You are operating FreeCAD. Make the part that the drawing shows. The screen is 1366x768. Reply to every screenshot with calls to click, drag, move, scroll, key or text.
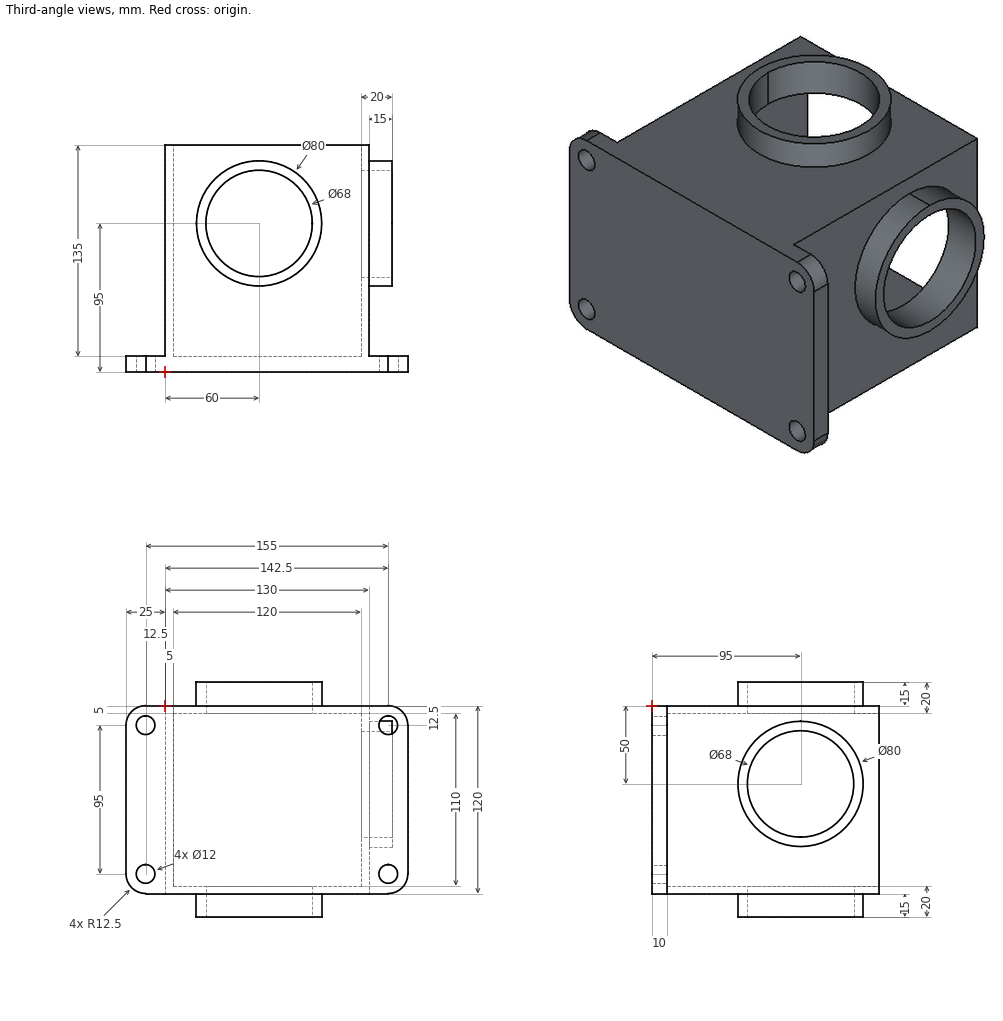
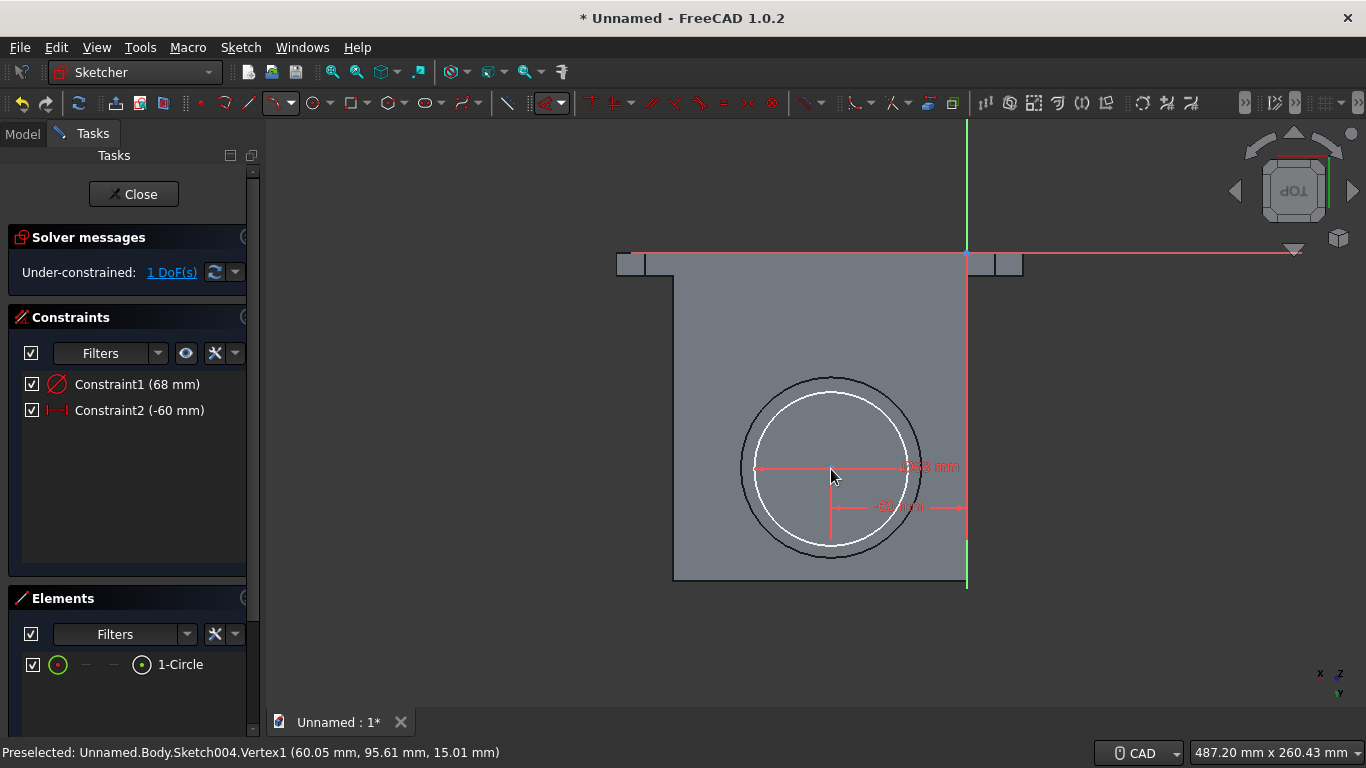
click(831, 469)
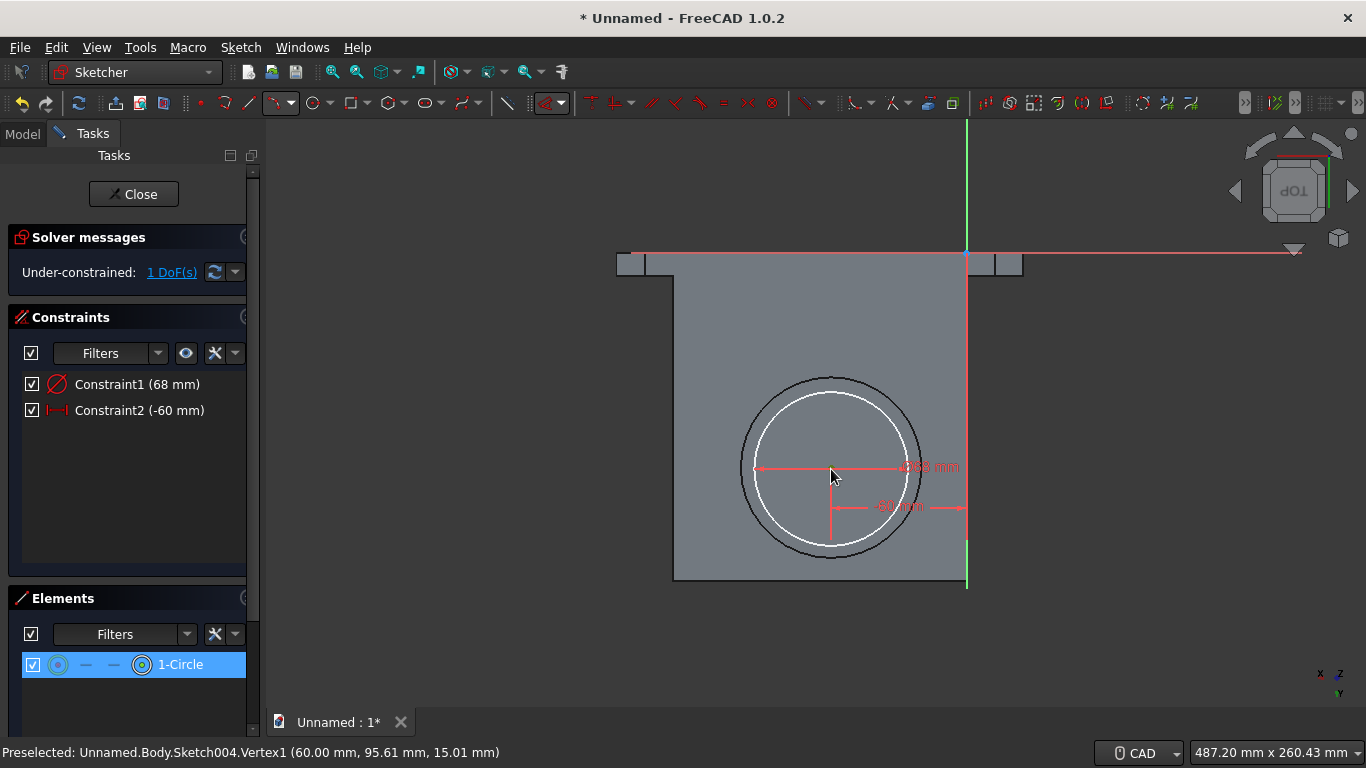
key(i)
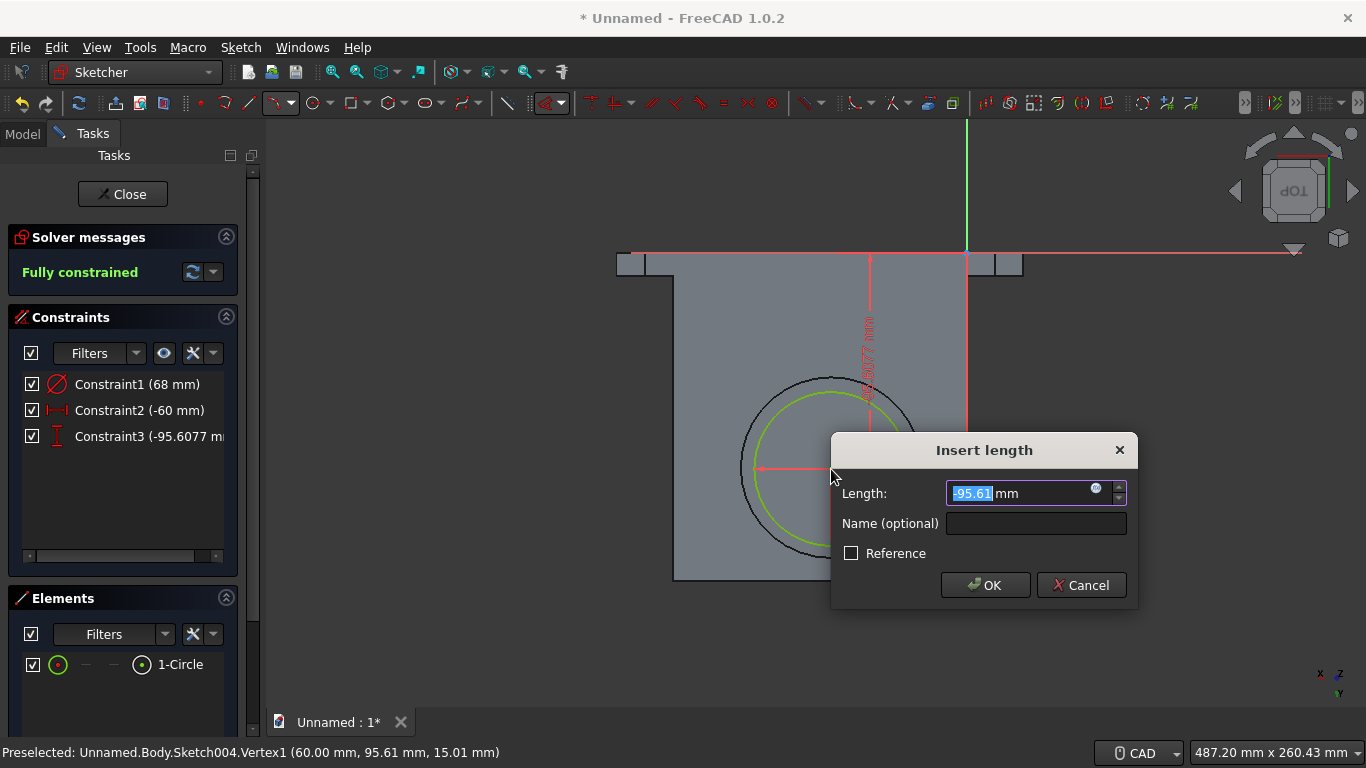
text(-95)
key(Return)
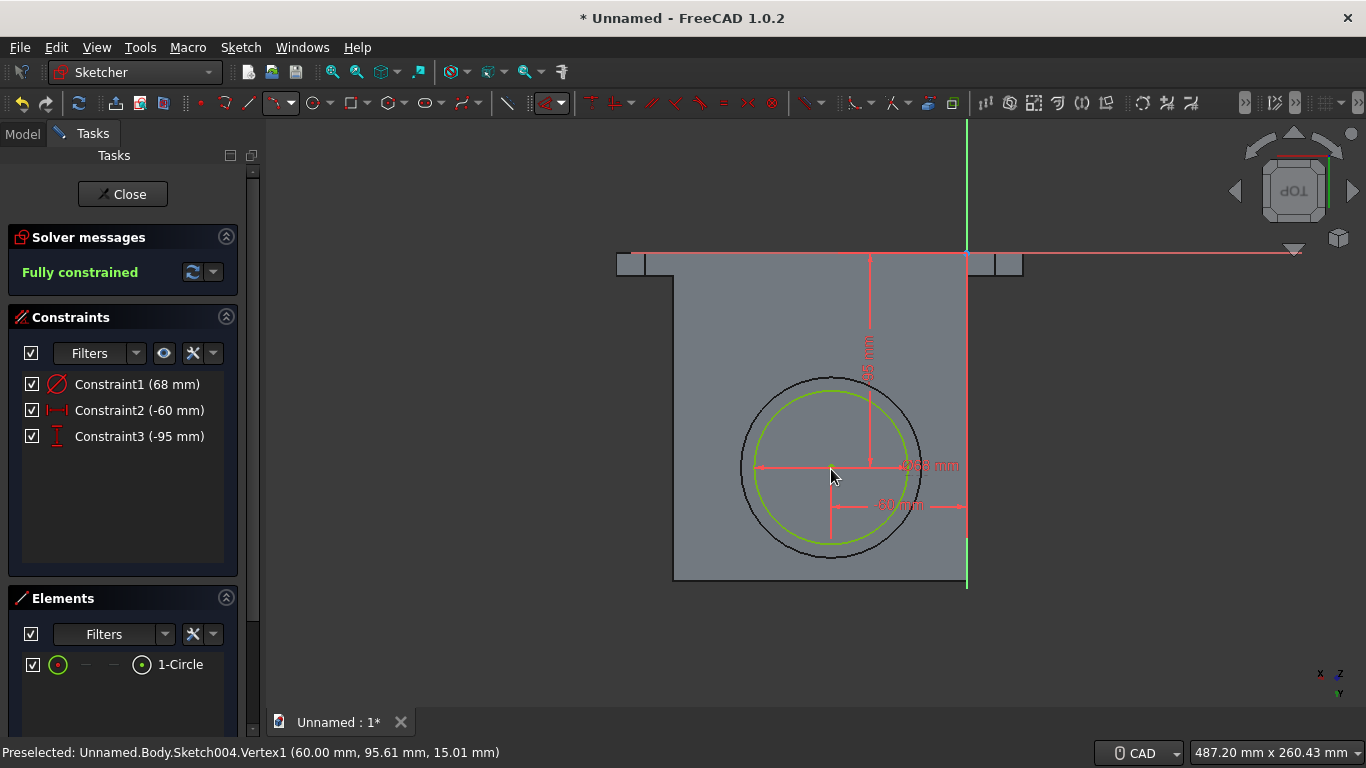
click(123, 194)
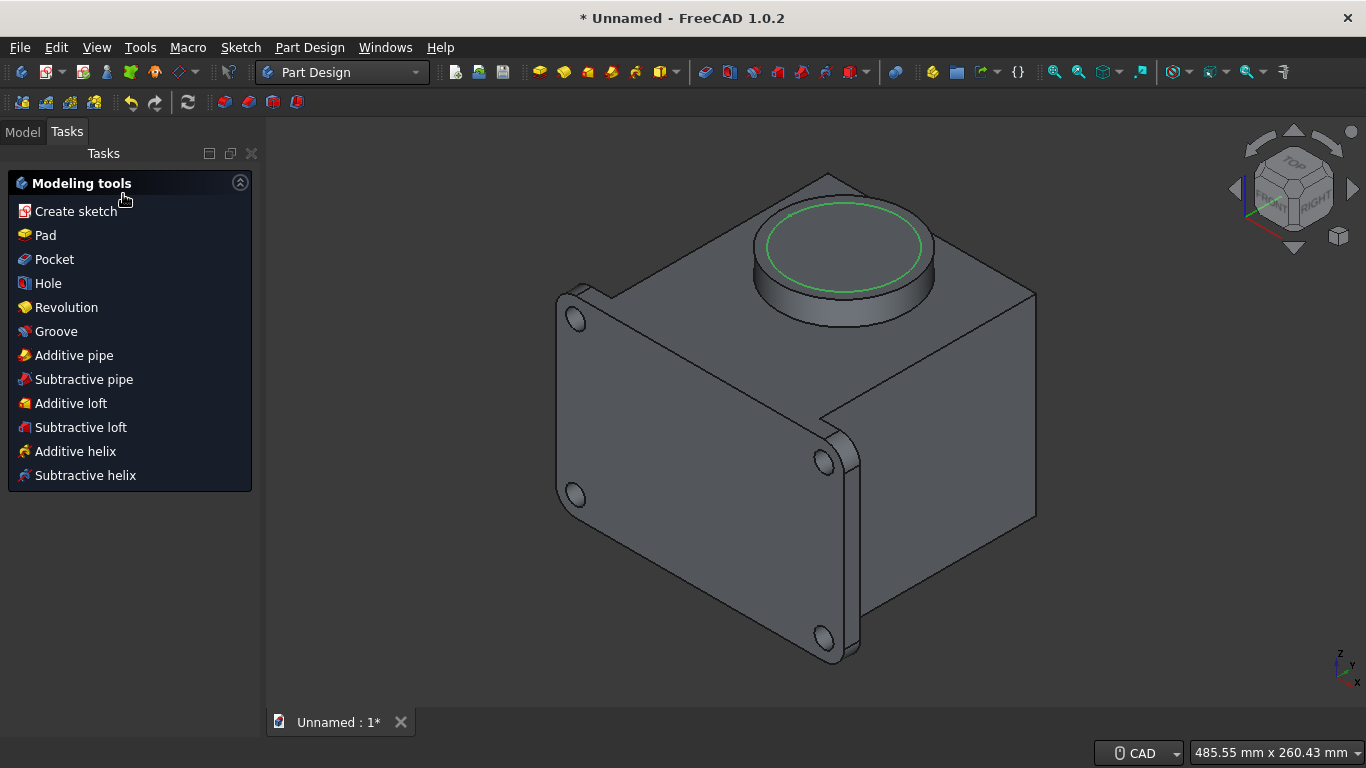
click(706, 72)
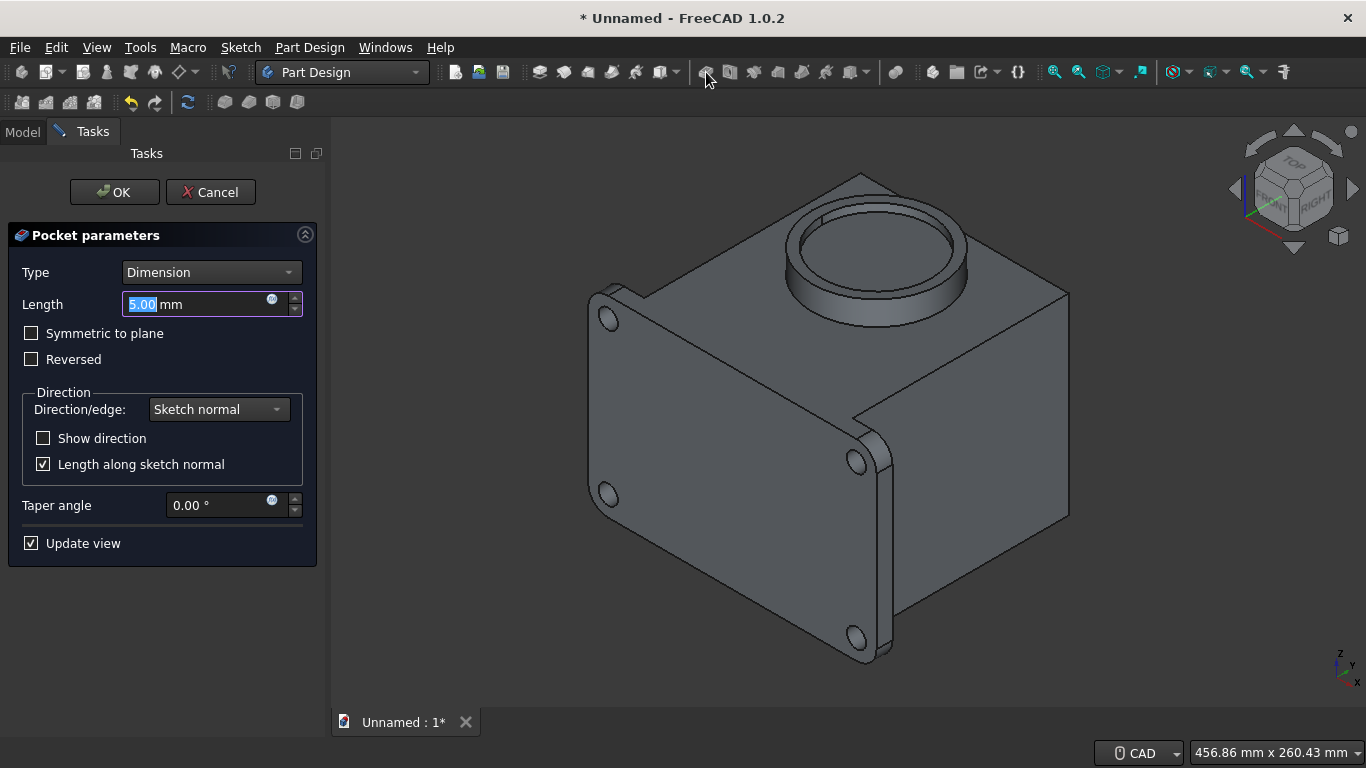
text(20)
key(Tab)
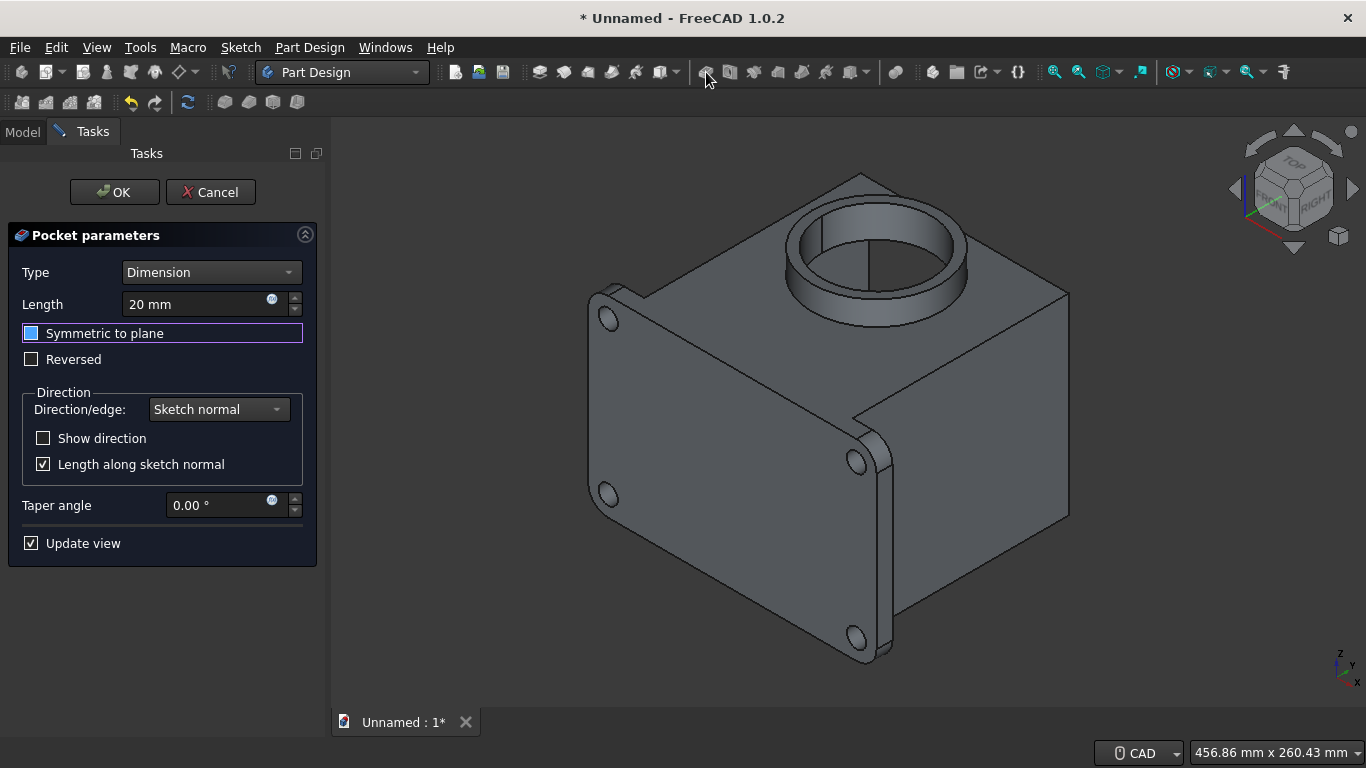
click(115, 192)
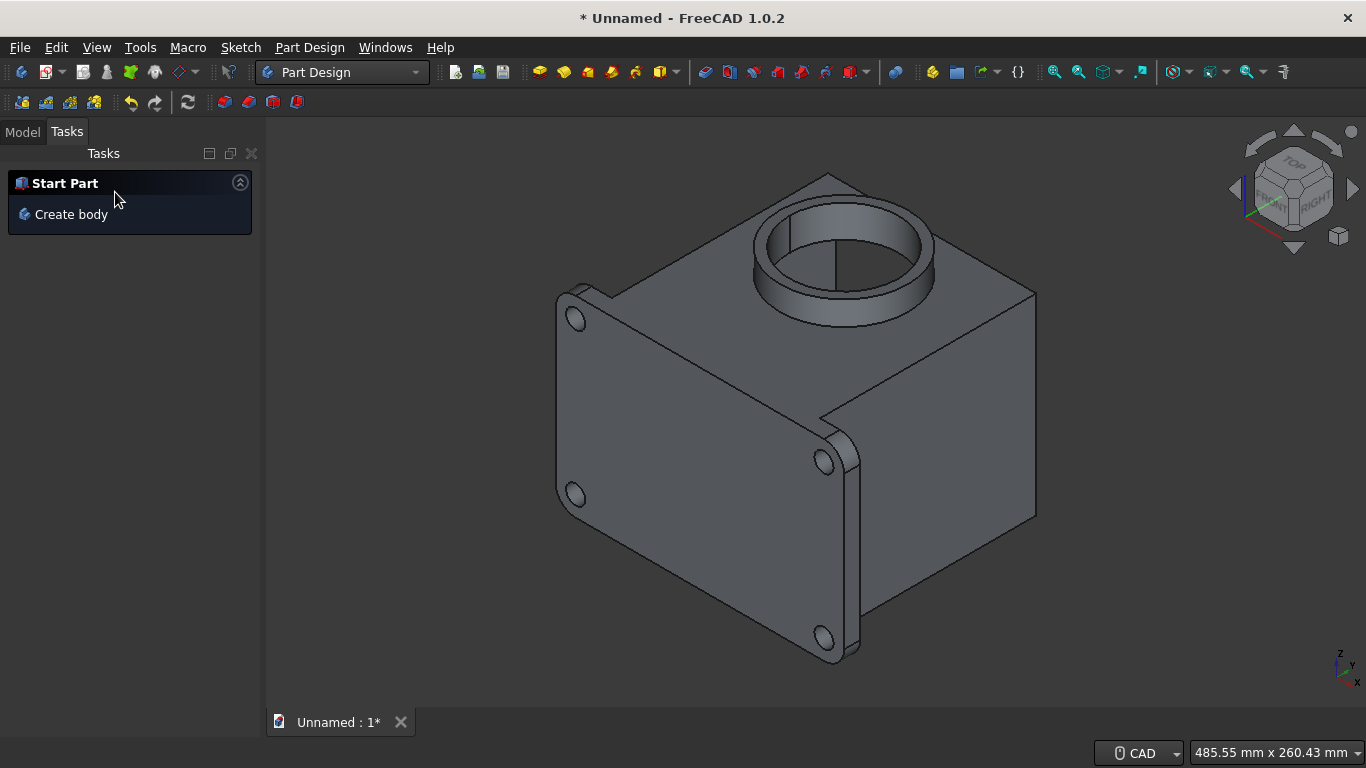
click(928, 466)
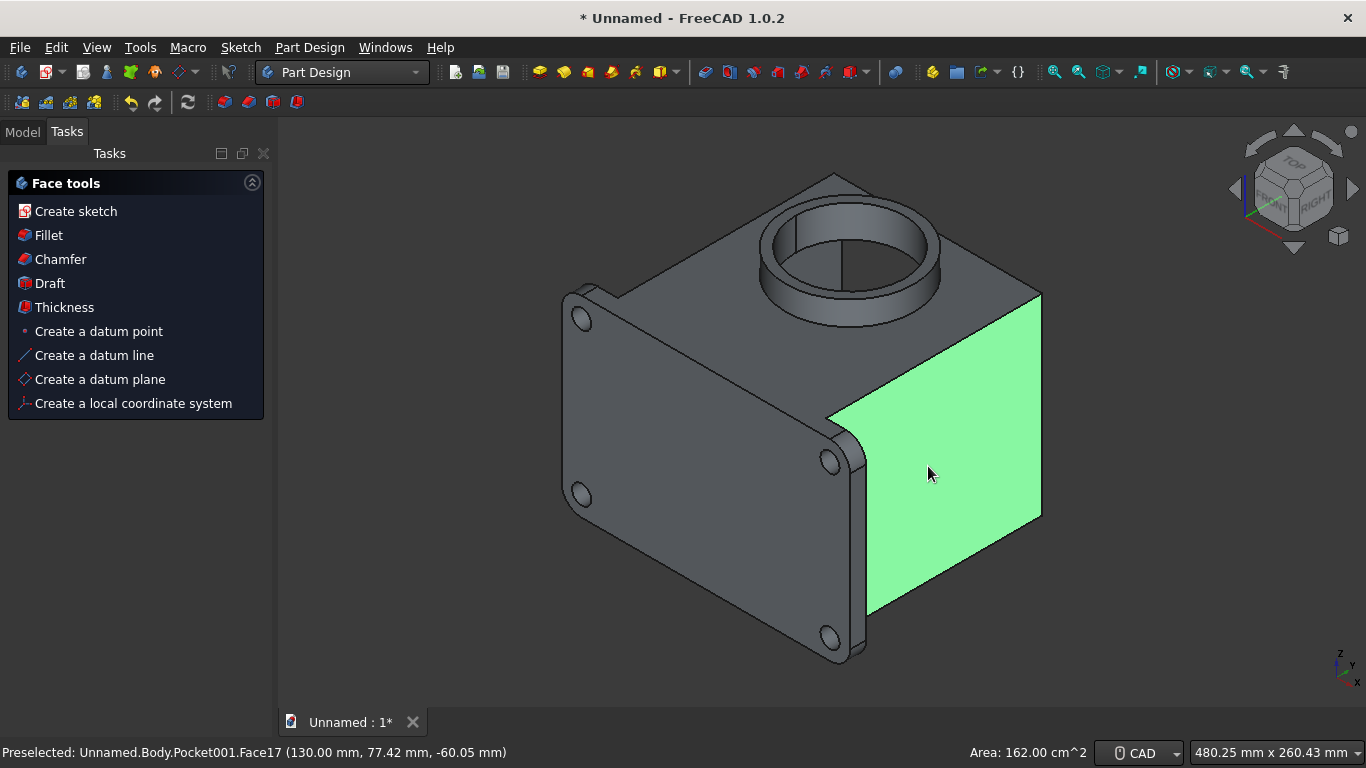
click(46, 72)